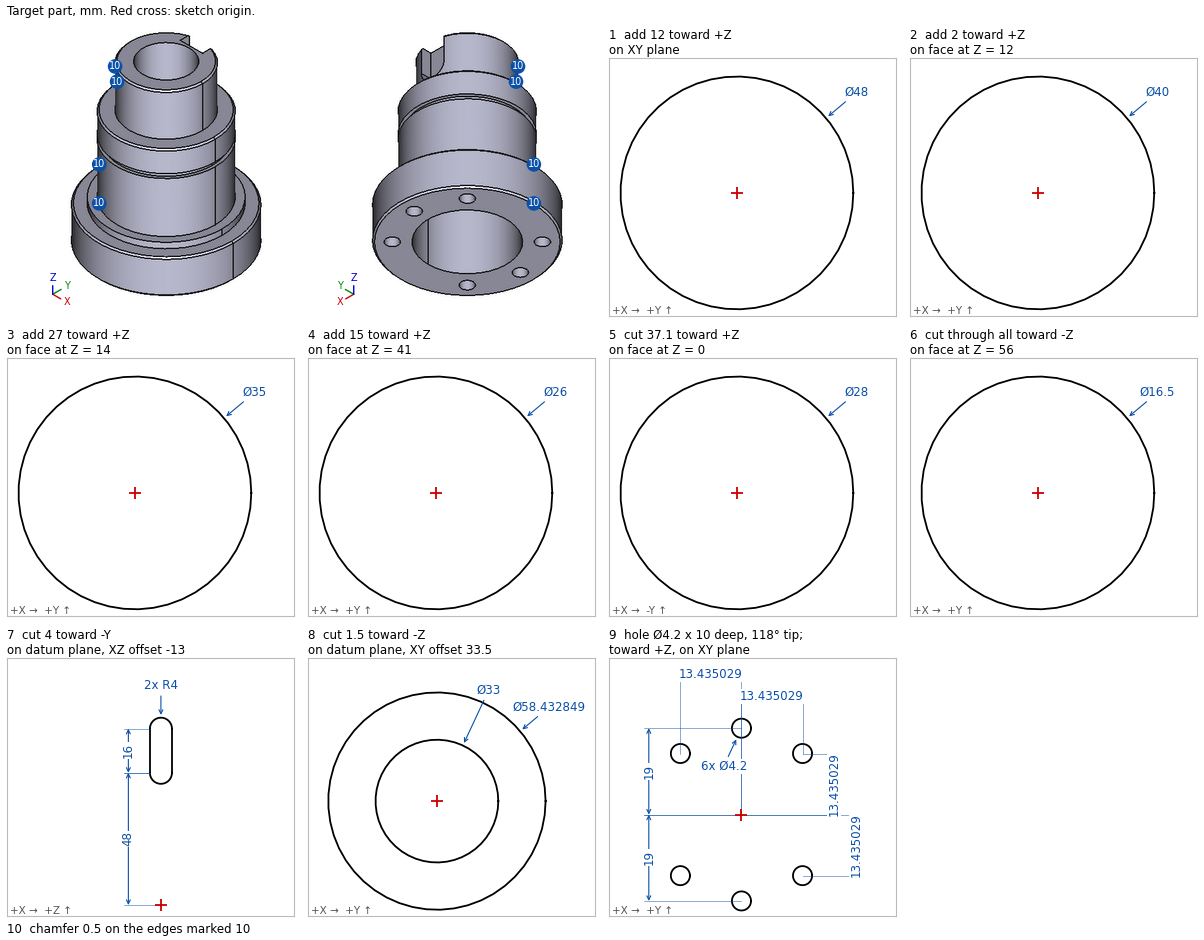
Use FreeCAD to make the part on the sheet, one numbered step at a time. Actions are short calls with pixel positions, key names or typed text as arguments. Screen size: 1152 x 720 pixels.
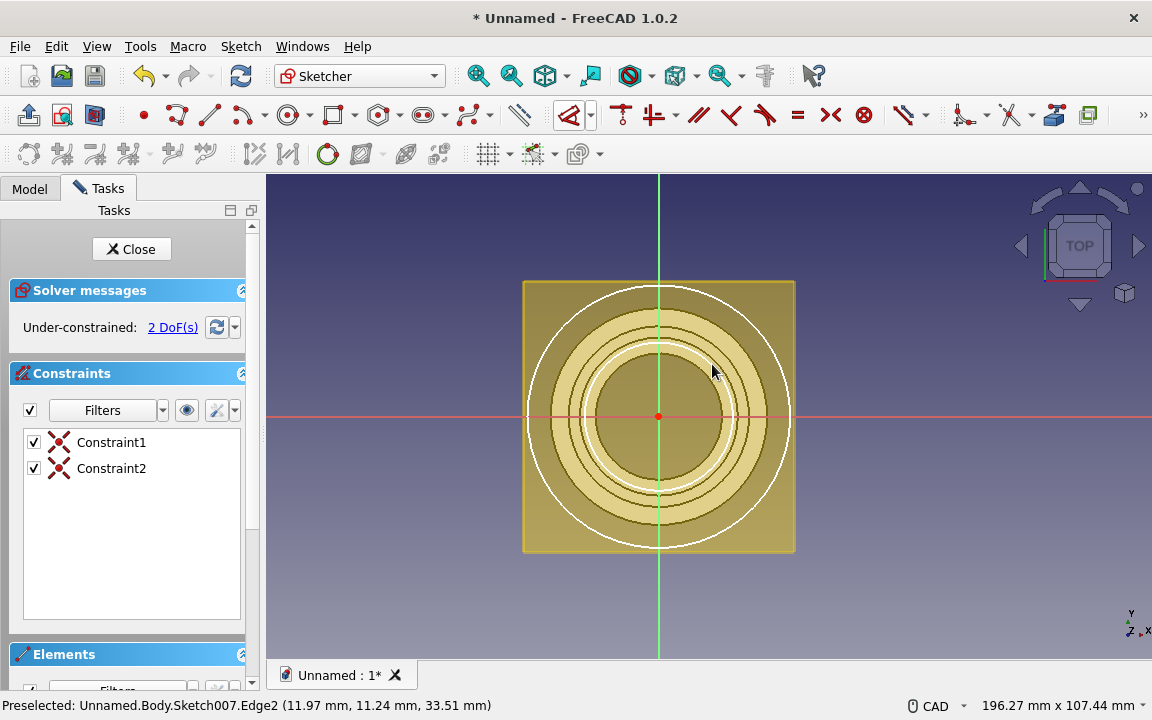
click(751, 323)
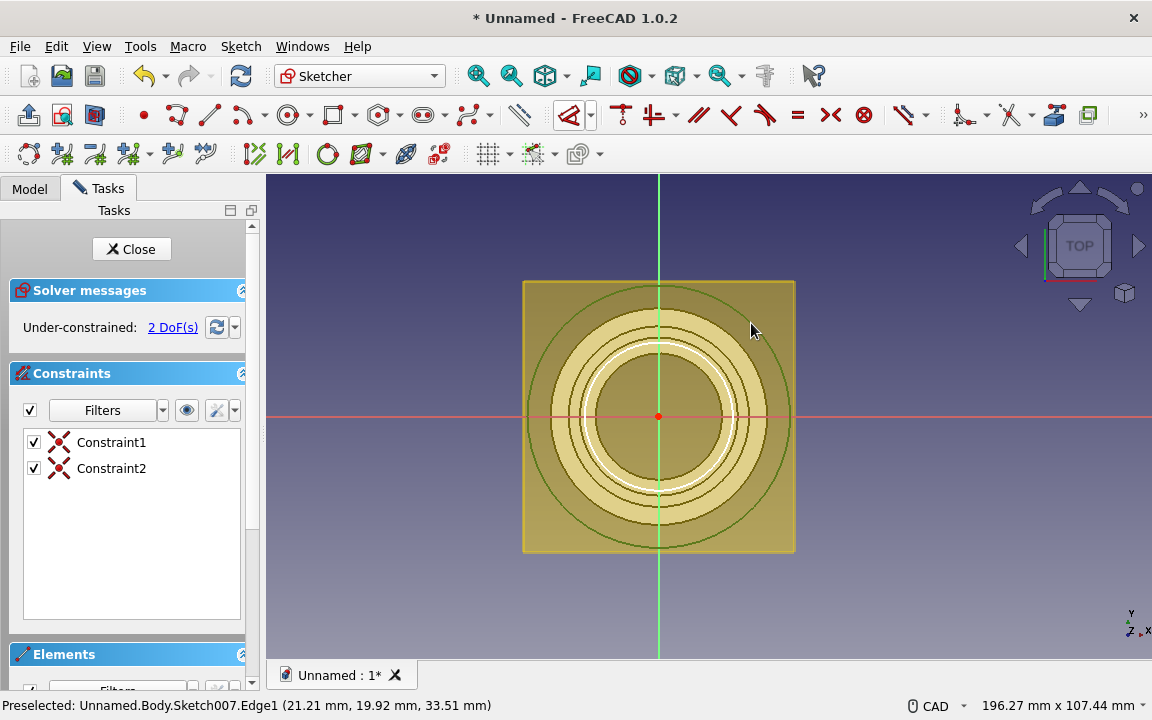
key(k)
key(o)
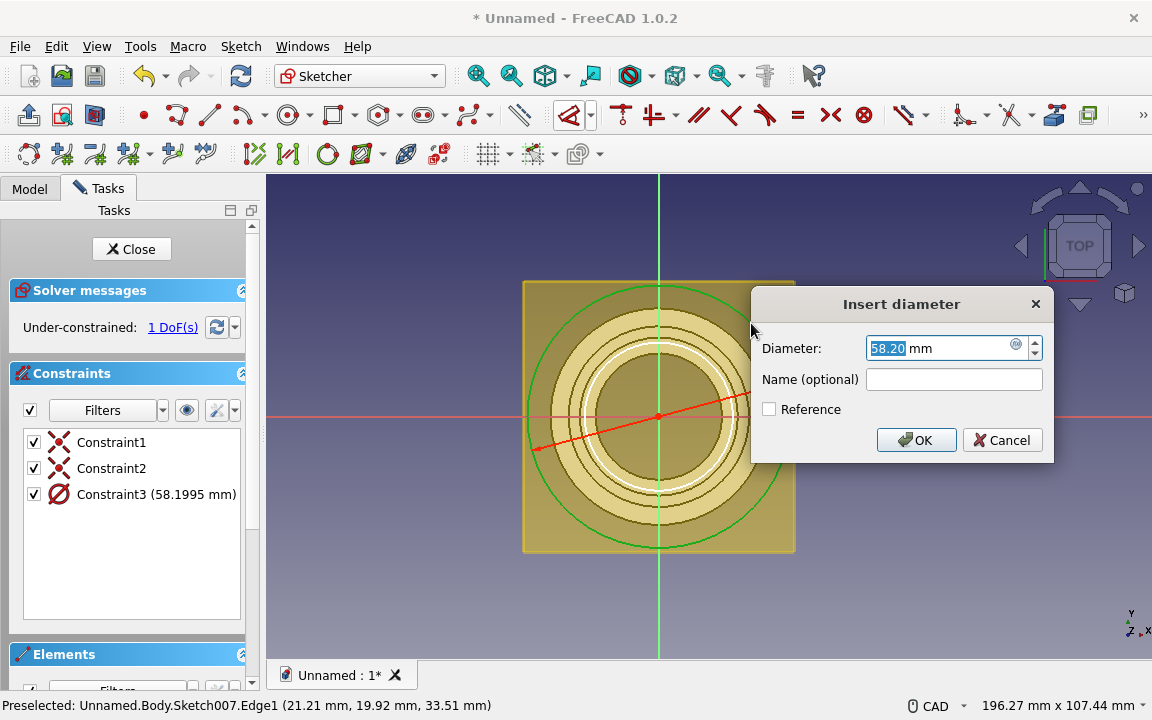
text(58.432849)
key(Return)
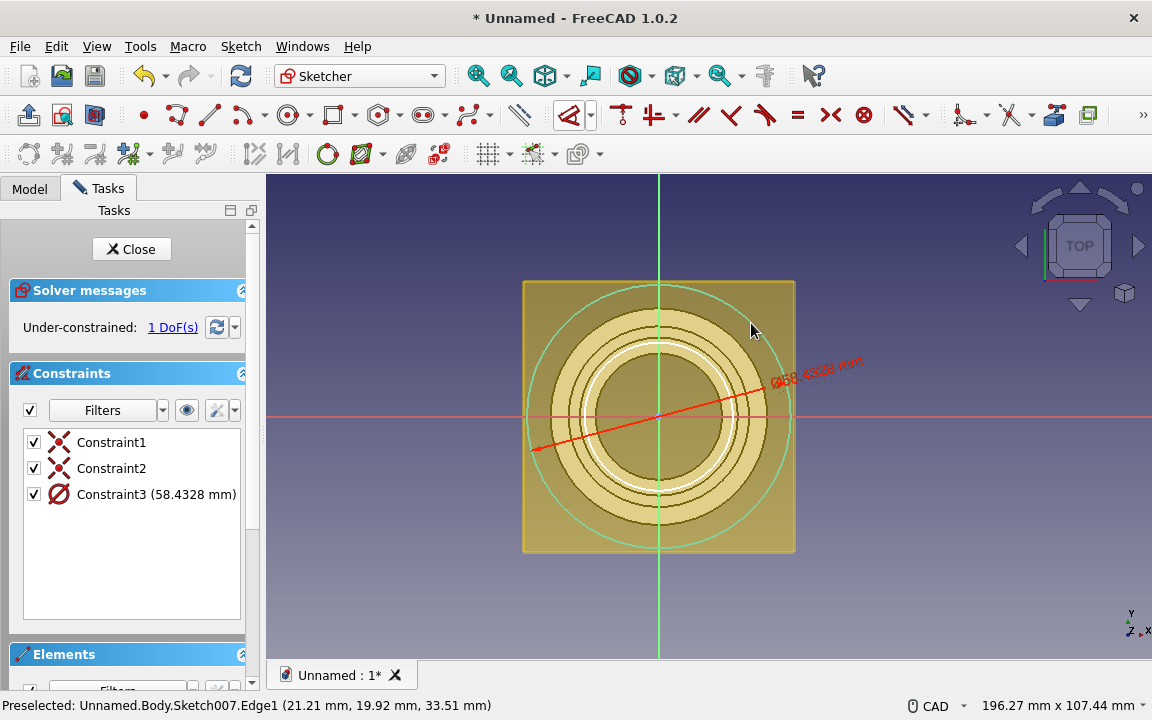
click(711, 364)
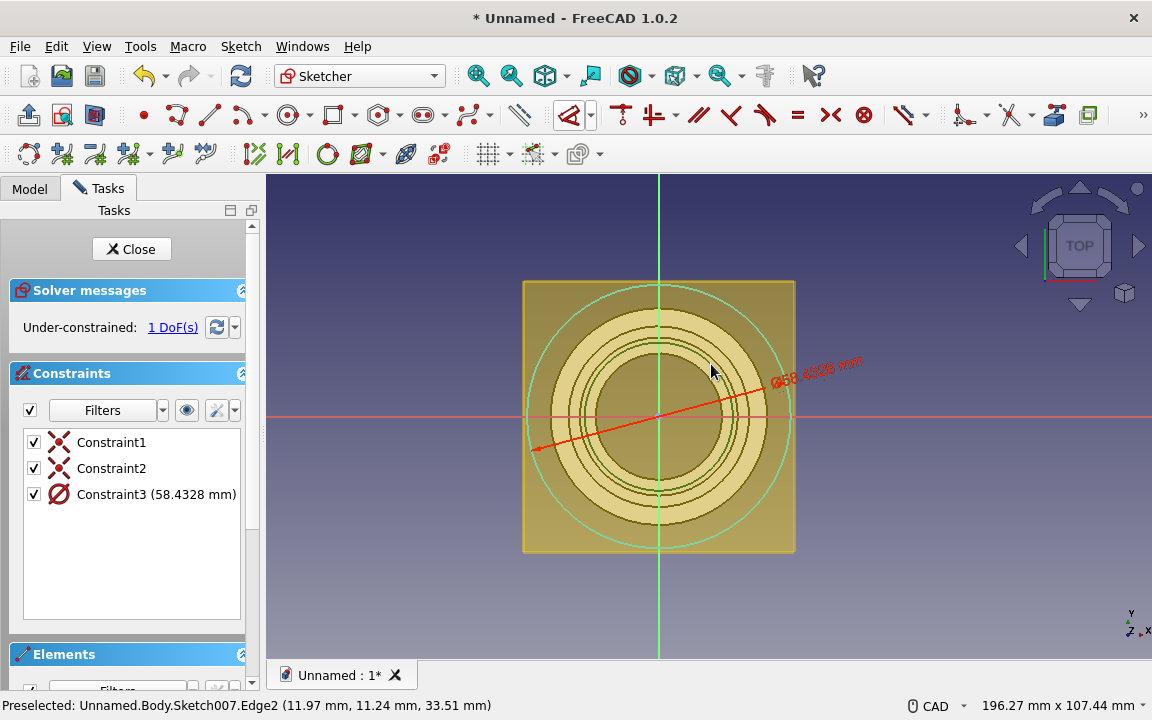
key(k)
key(o)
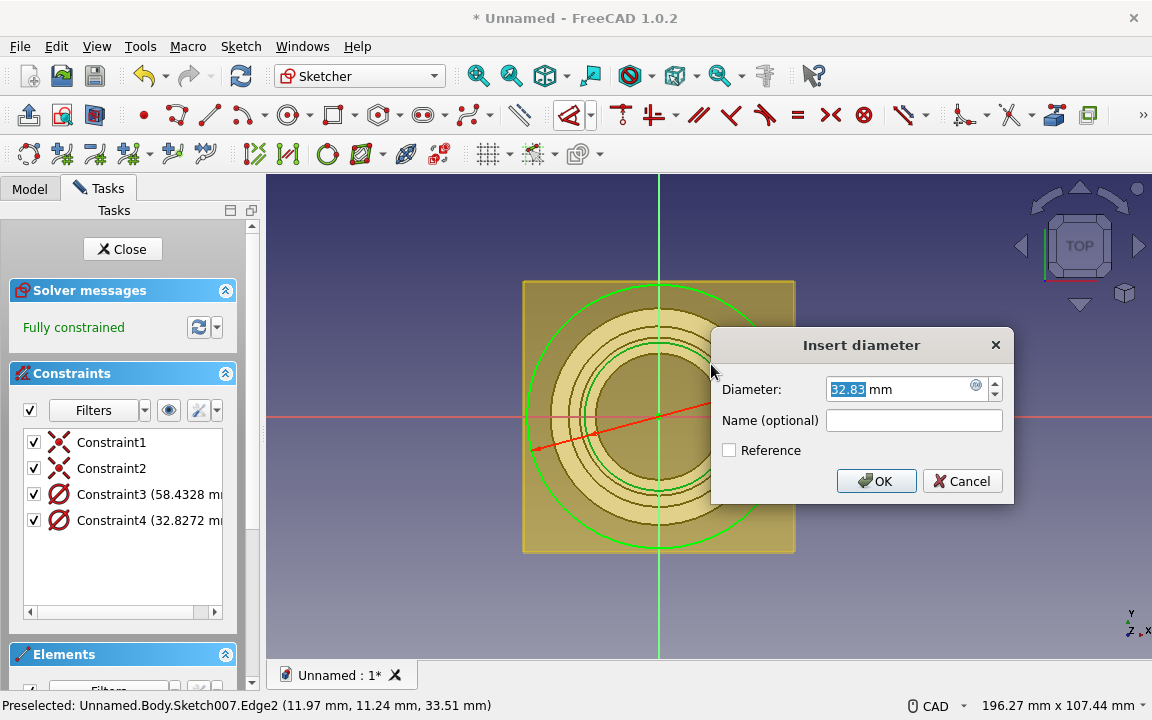
text(33)
key(Return)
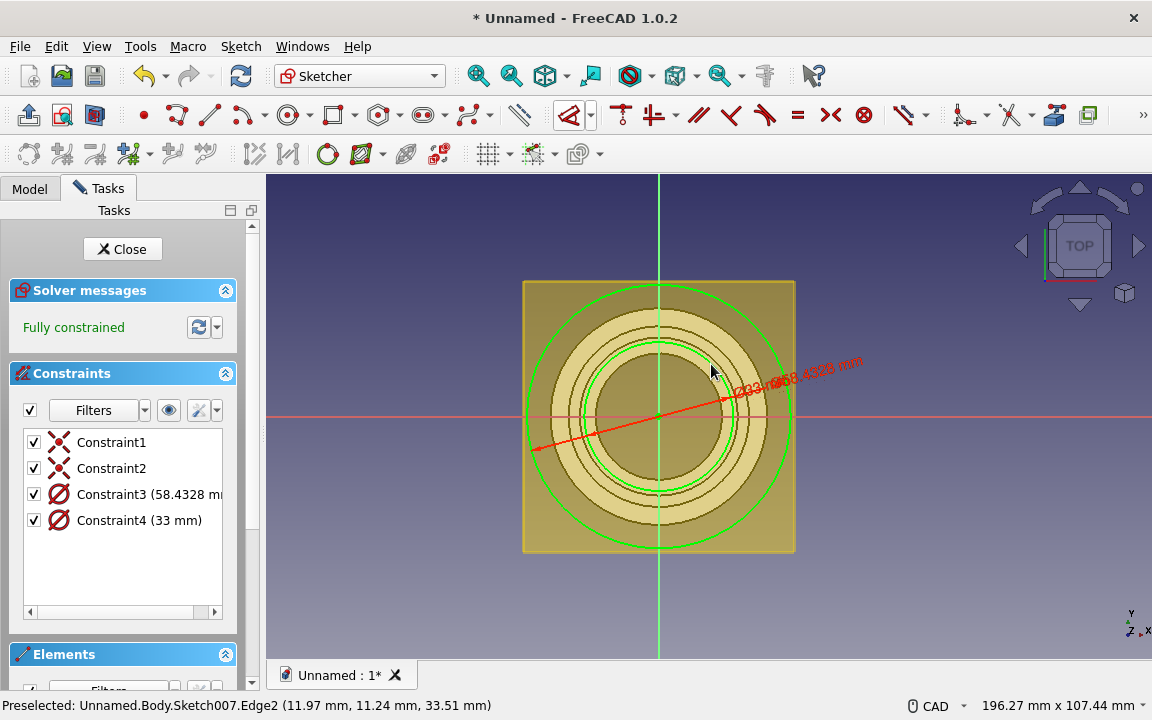
click(123, 249)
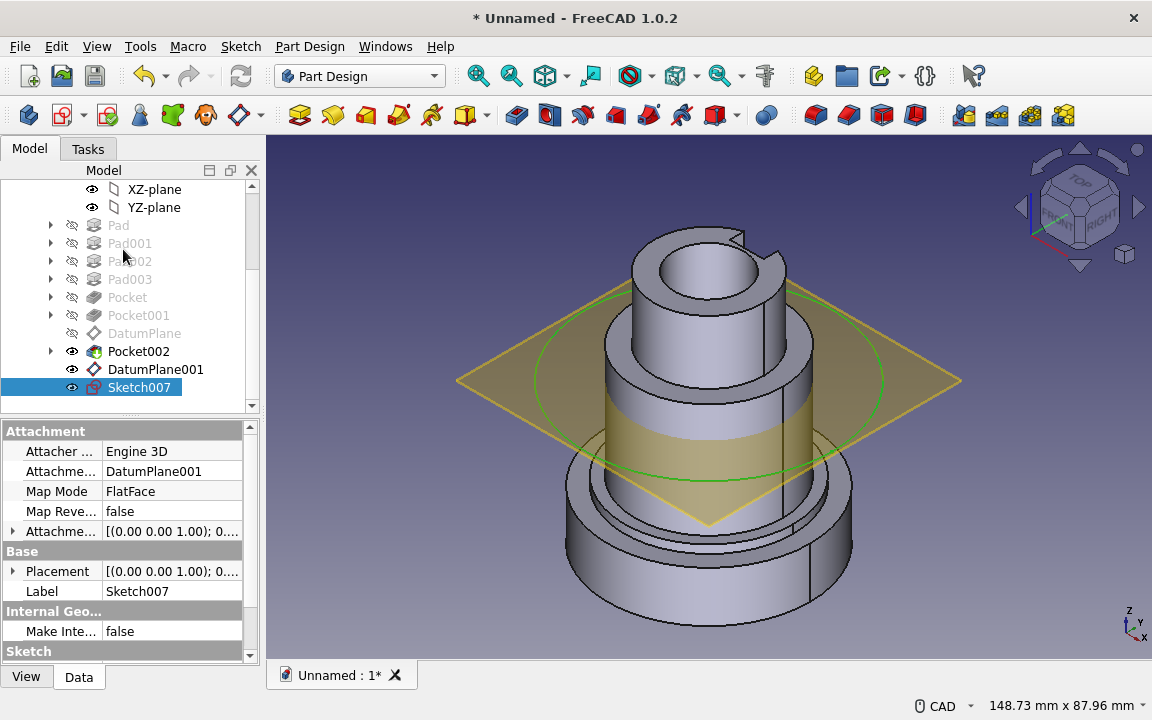
click(517, 116)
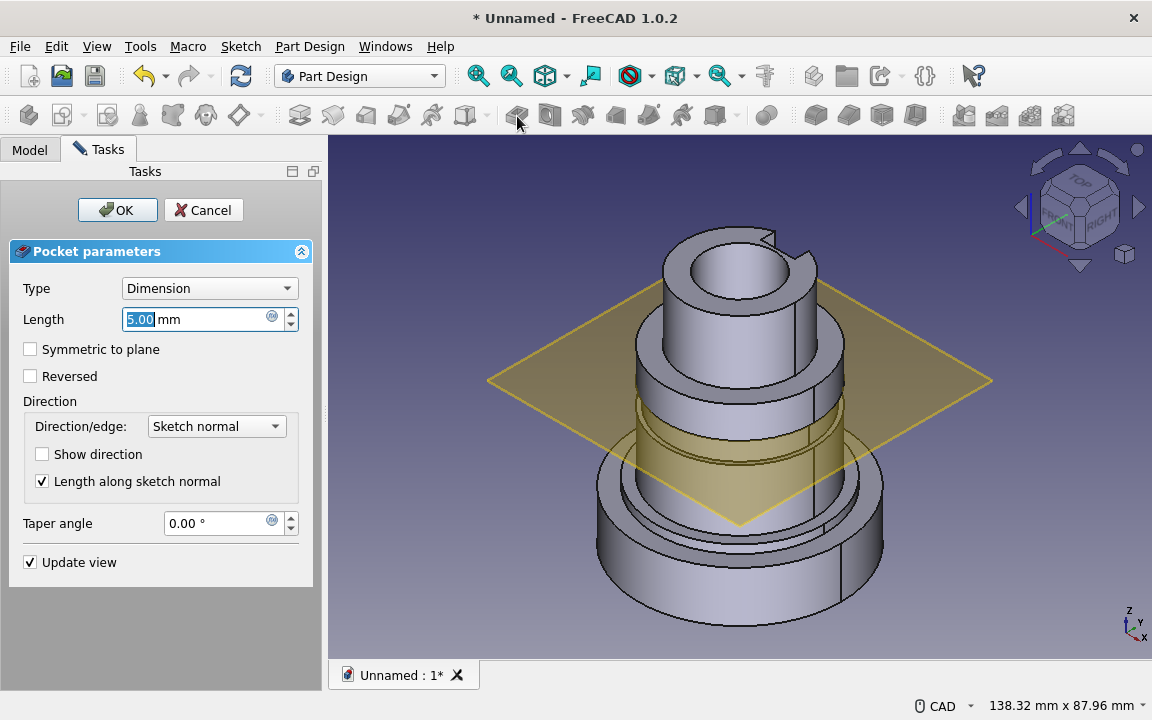
text(1.5)
key(Tab)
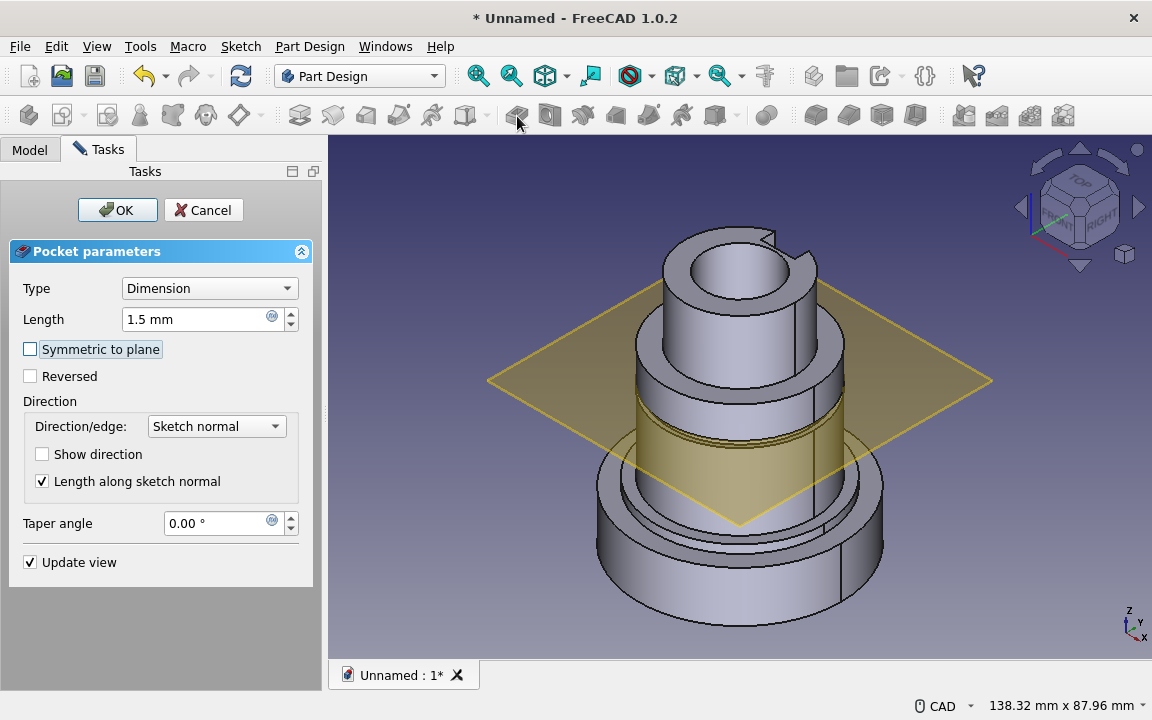
click(118, 210)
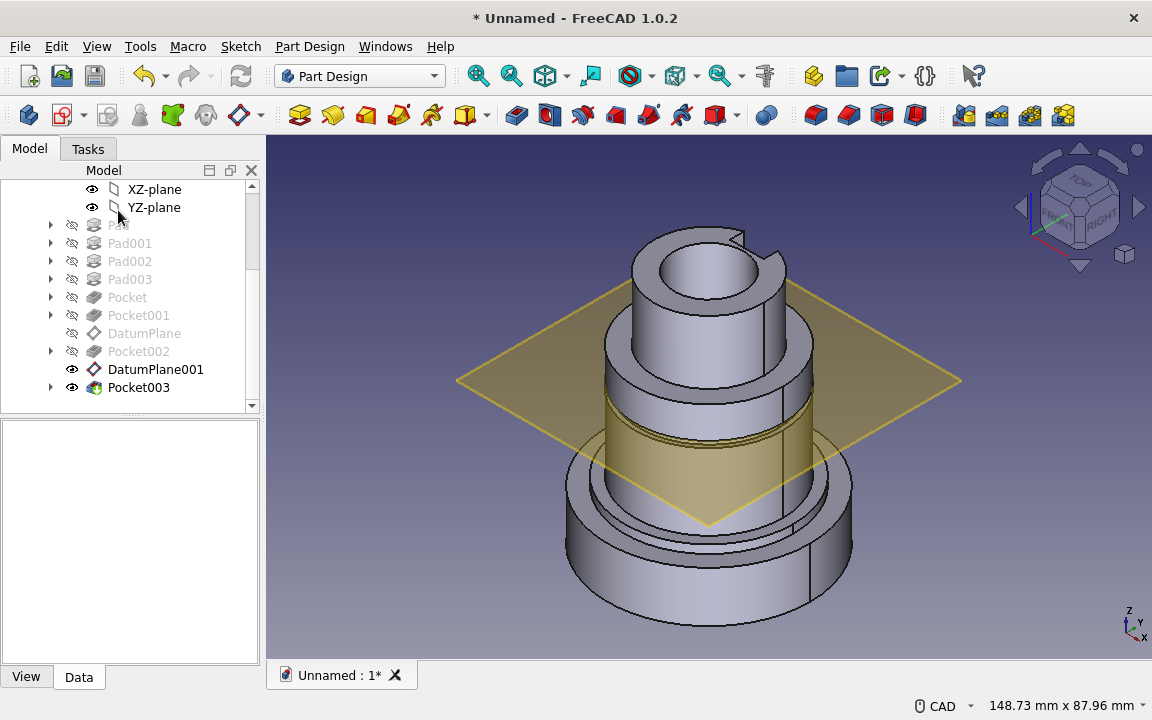
click(117, 369)
key(space)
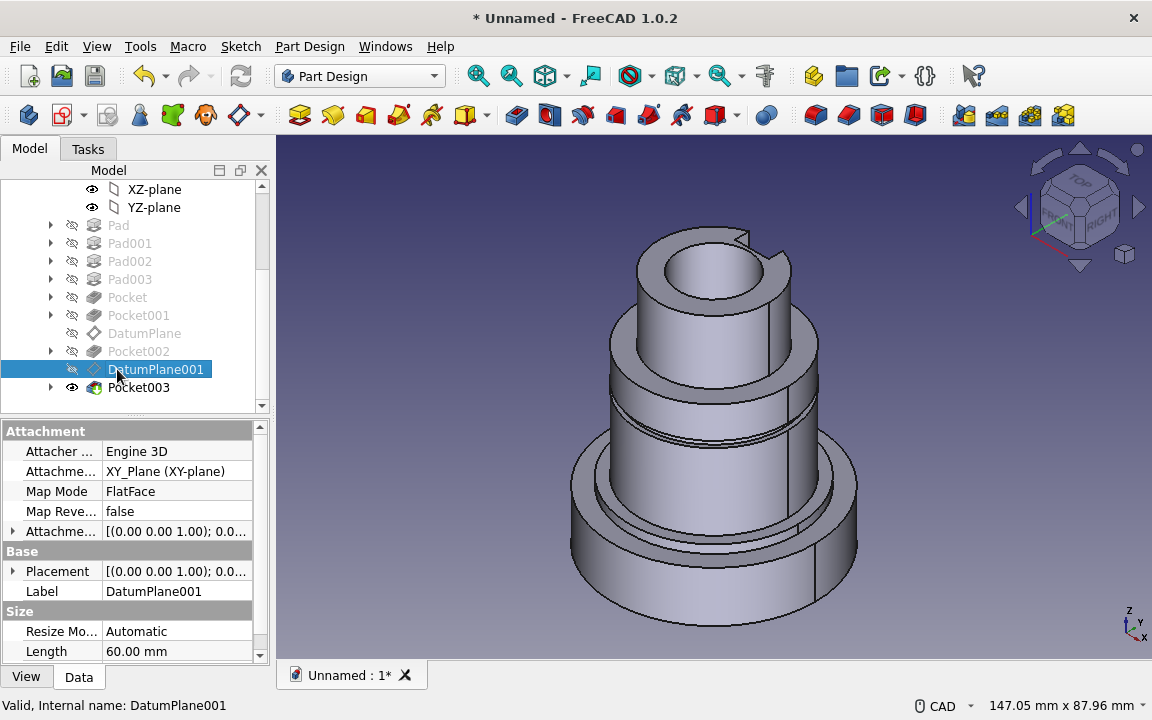
click(316, 619)